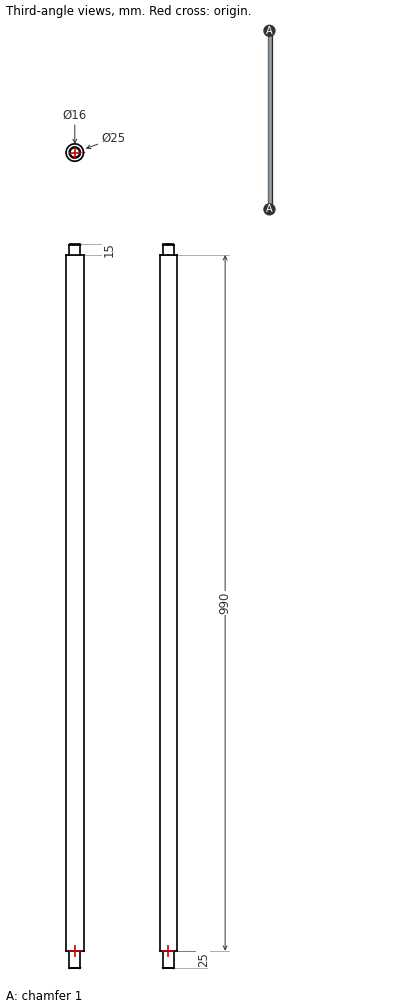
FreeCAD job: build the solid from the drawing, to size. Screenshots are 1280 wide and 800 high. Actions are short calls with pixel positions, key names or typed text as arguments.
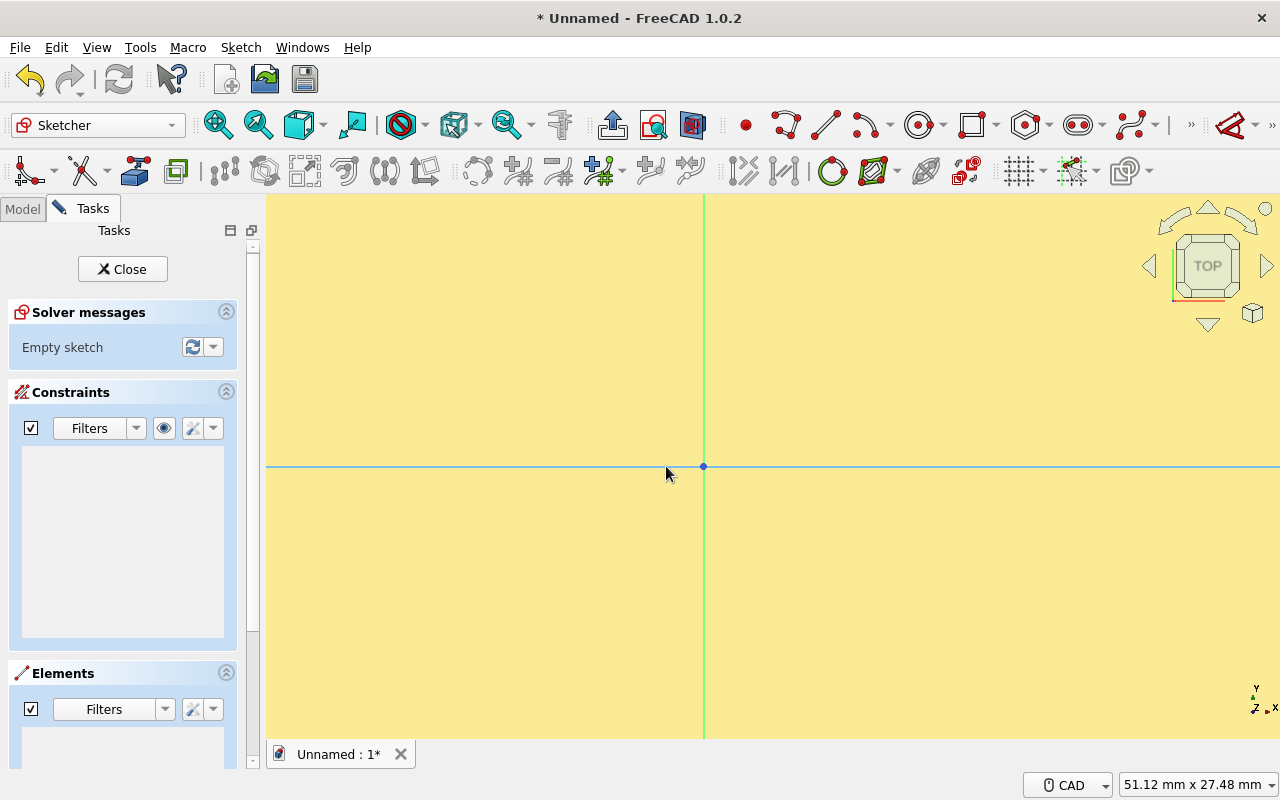
click(920, 126)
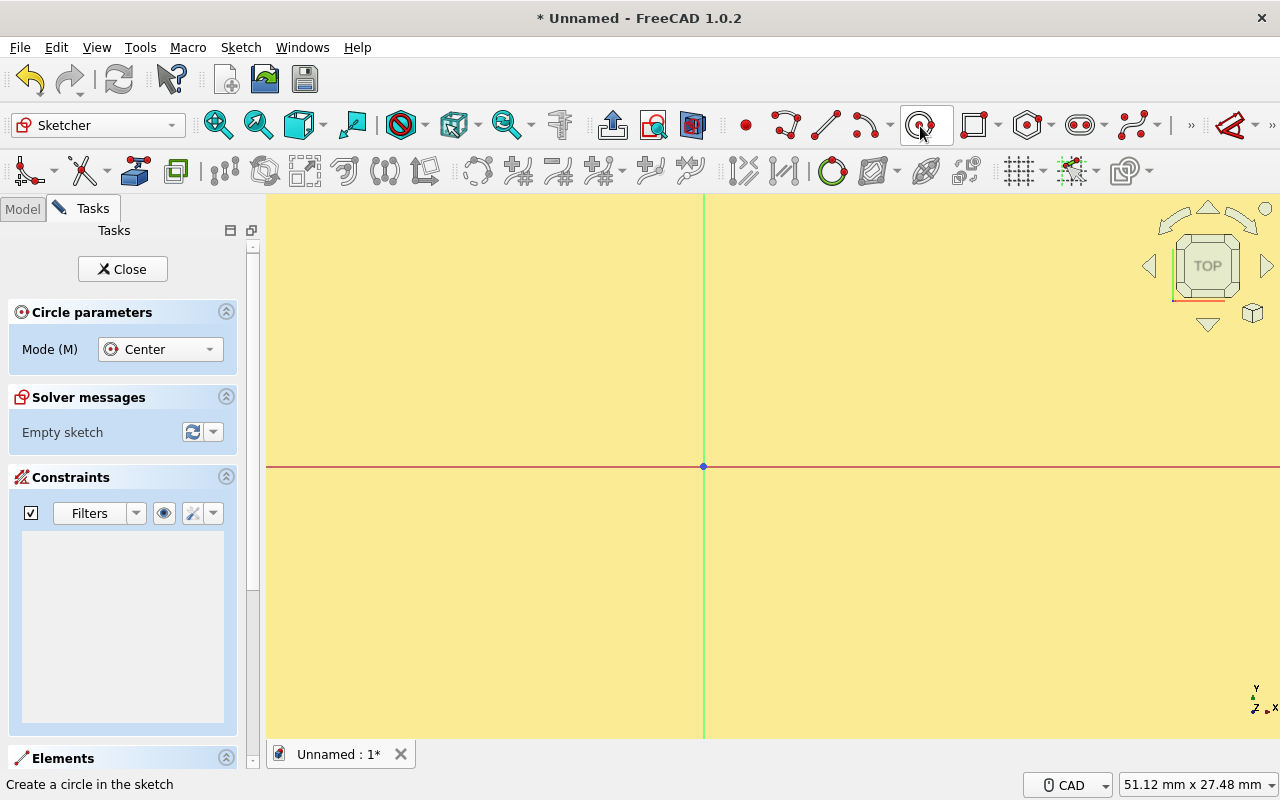
click(704, 466)
move(816, 354)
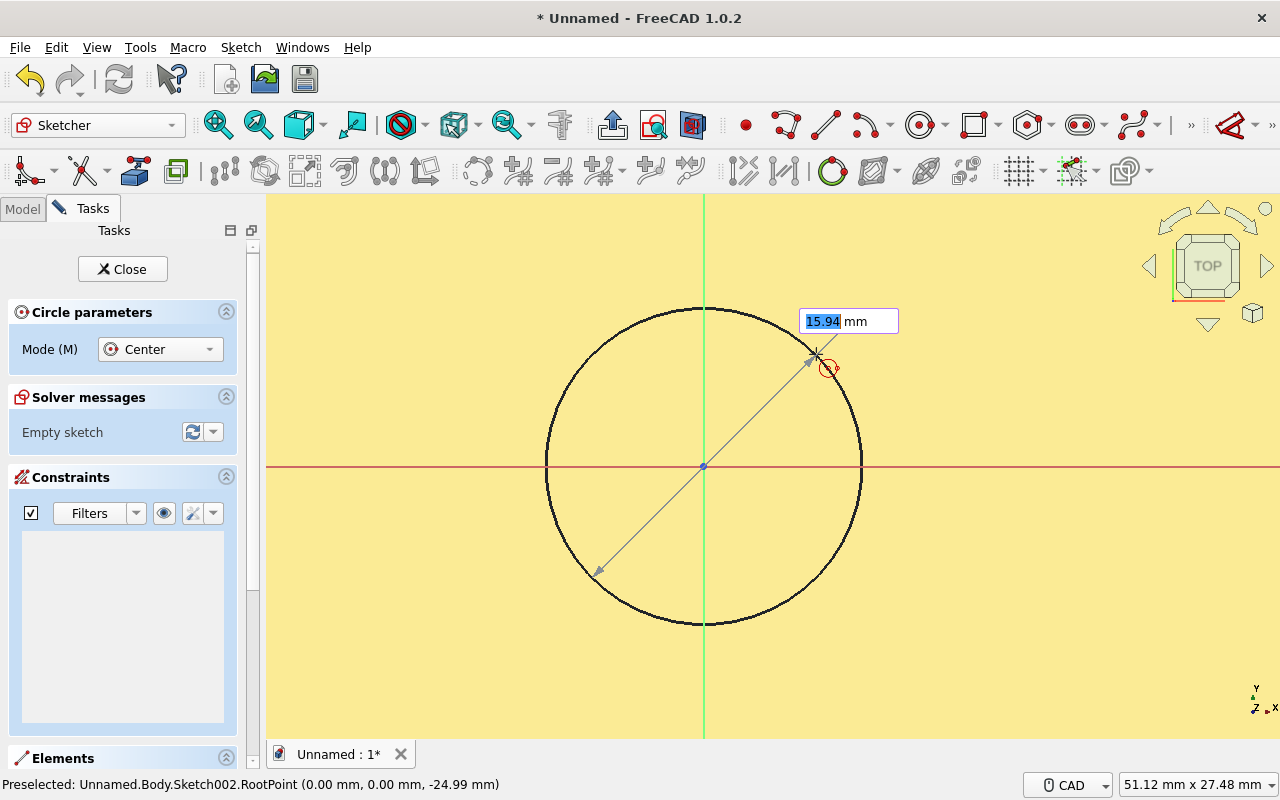
text(16)
key(Return)
key(Escape)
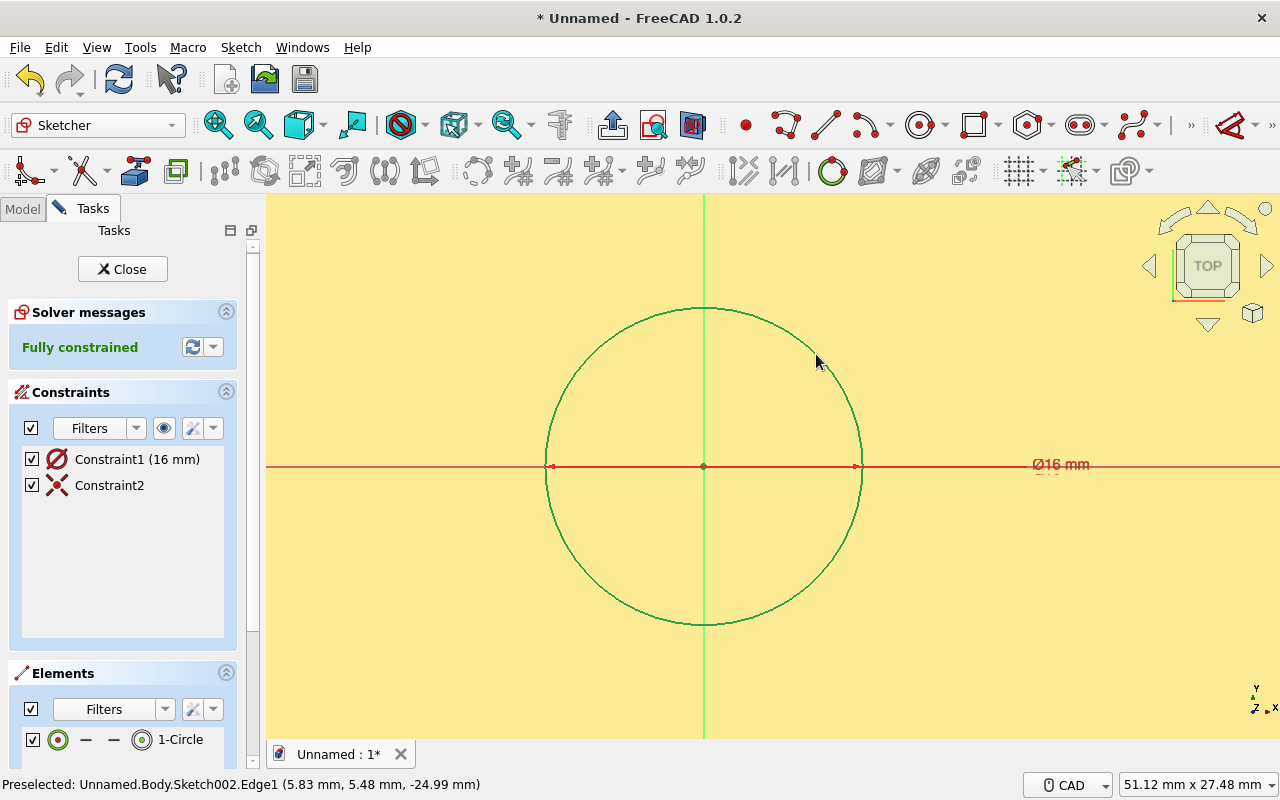
click(123, 269)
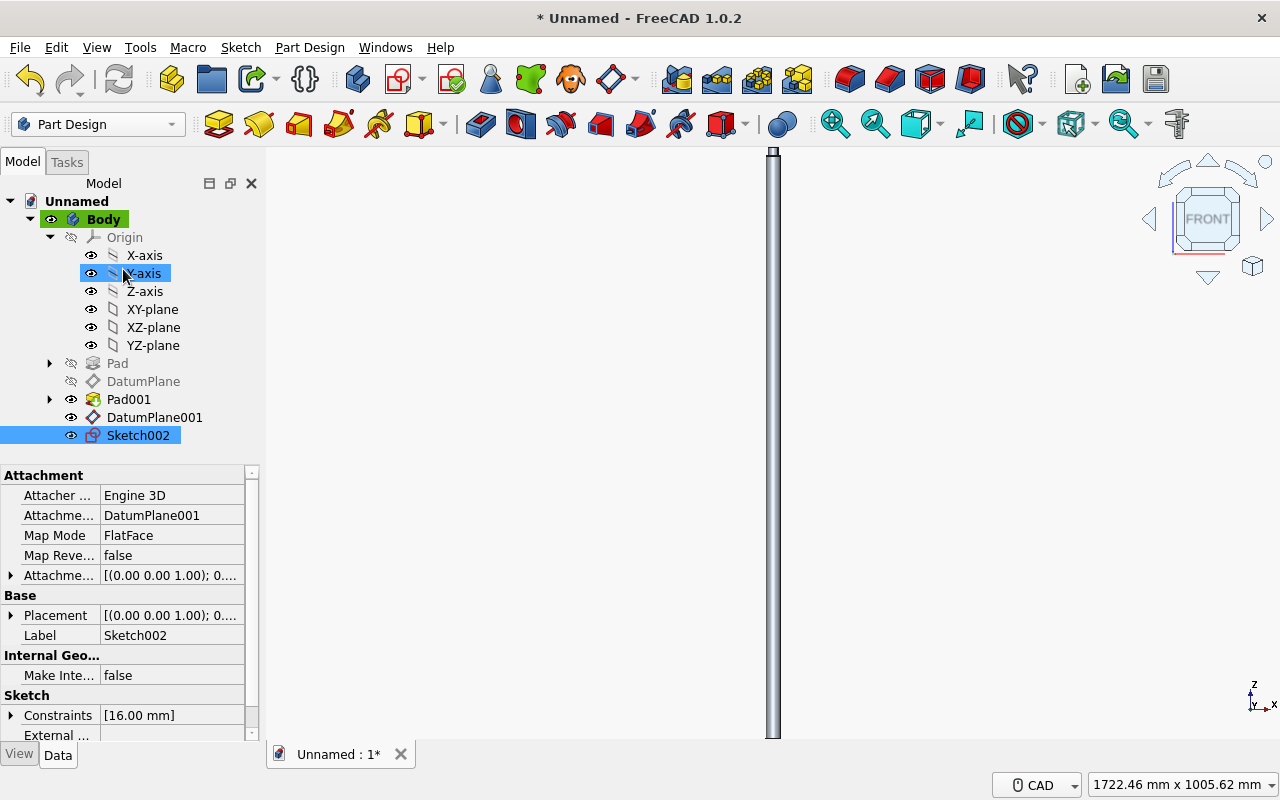
click(220, 124)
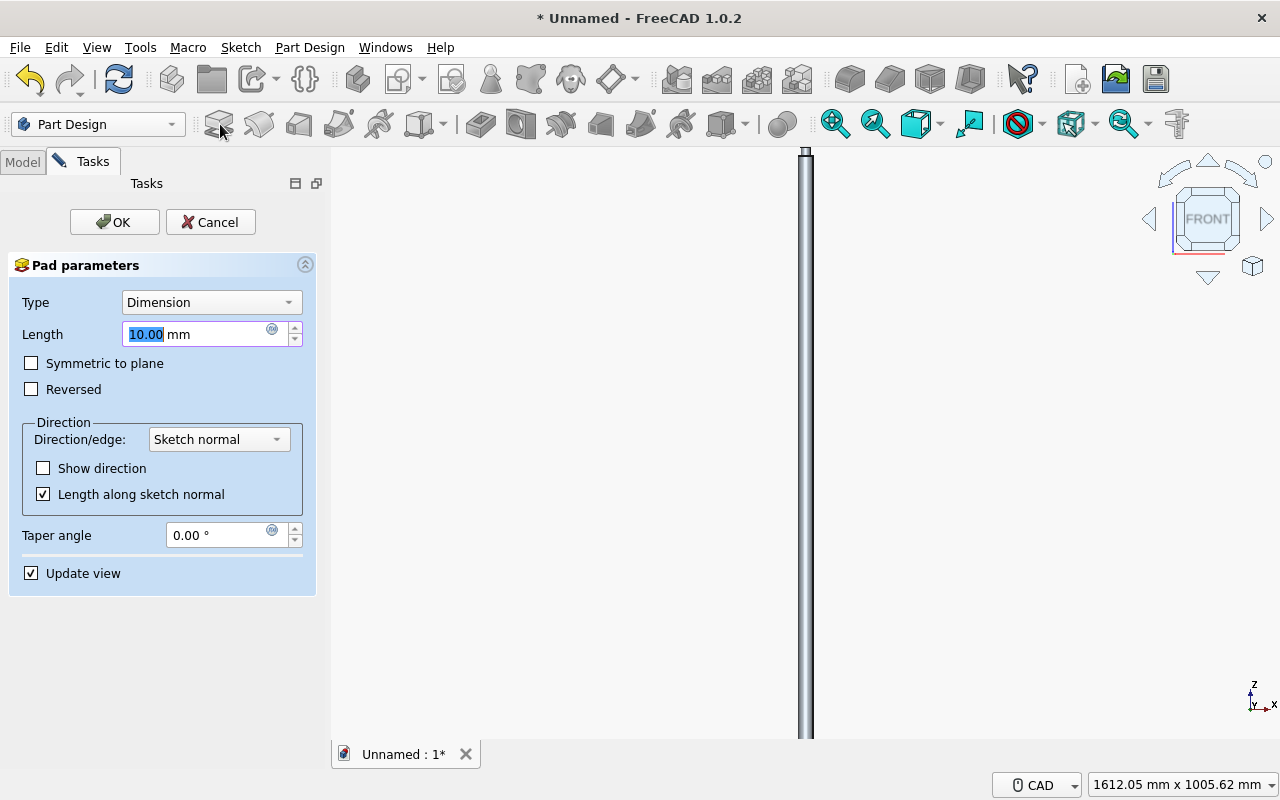
text(25)
key(Tab)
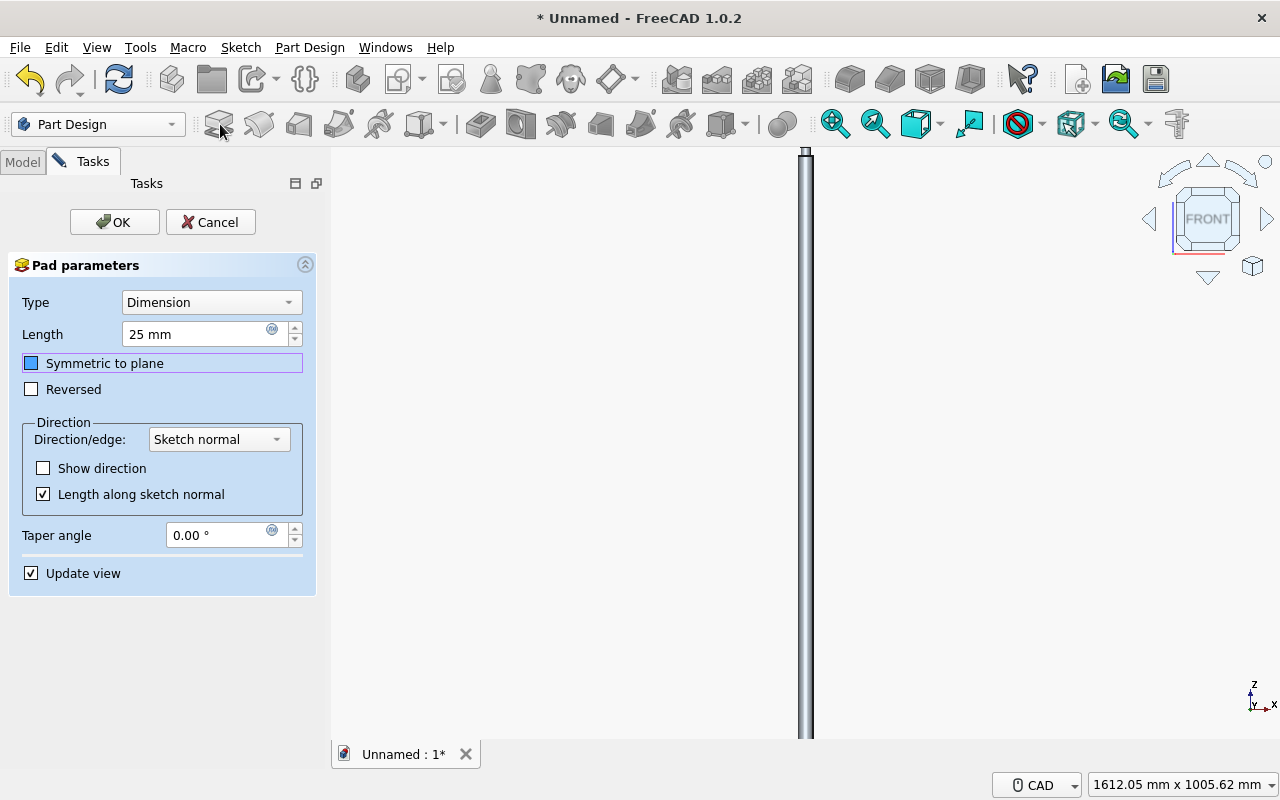
click(115, 222)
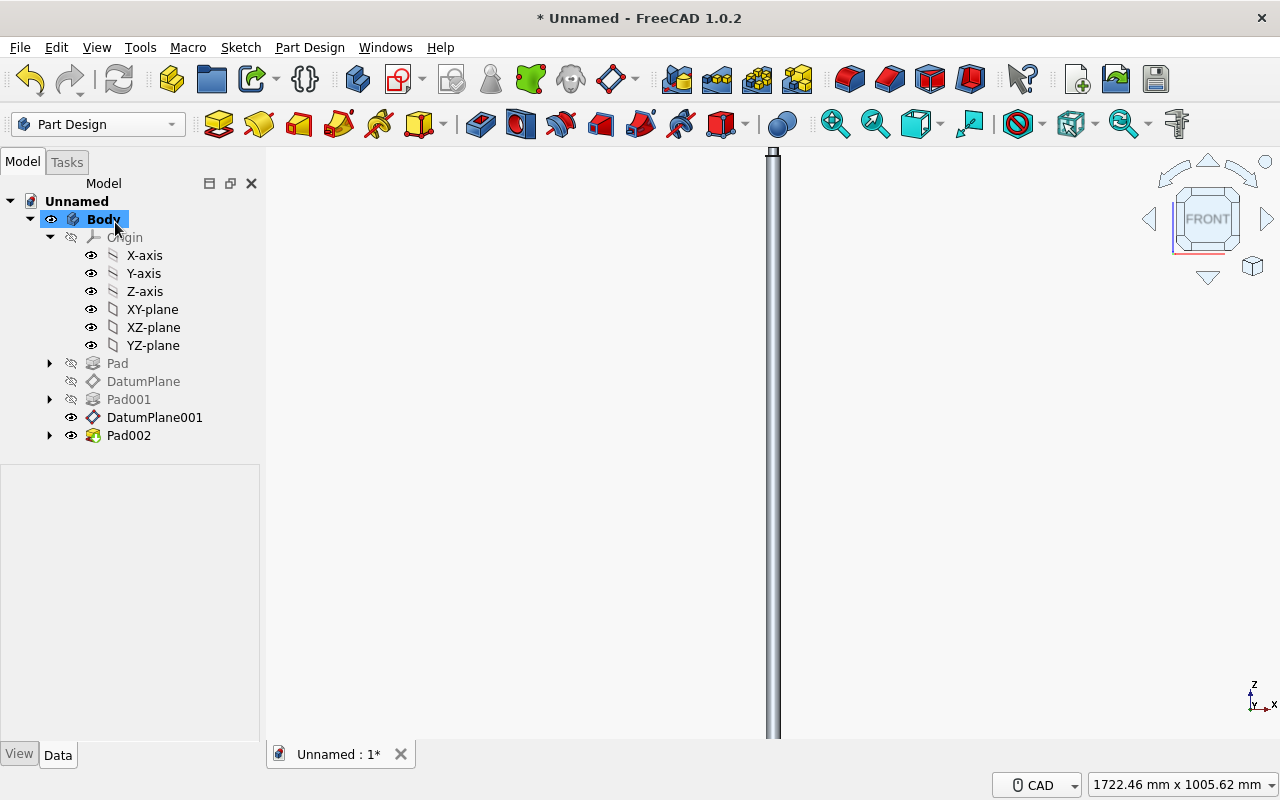
click(116, 417)
key(space)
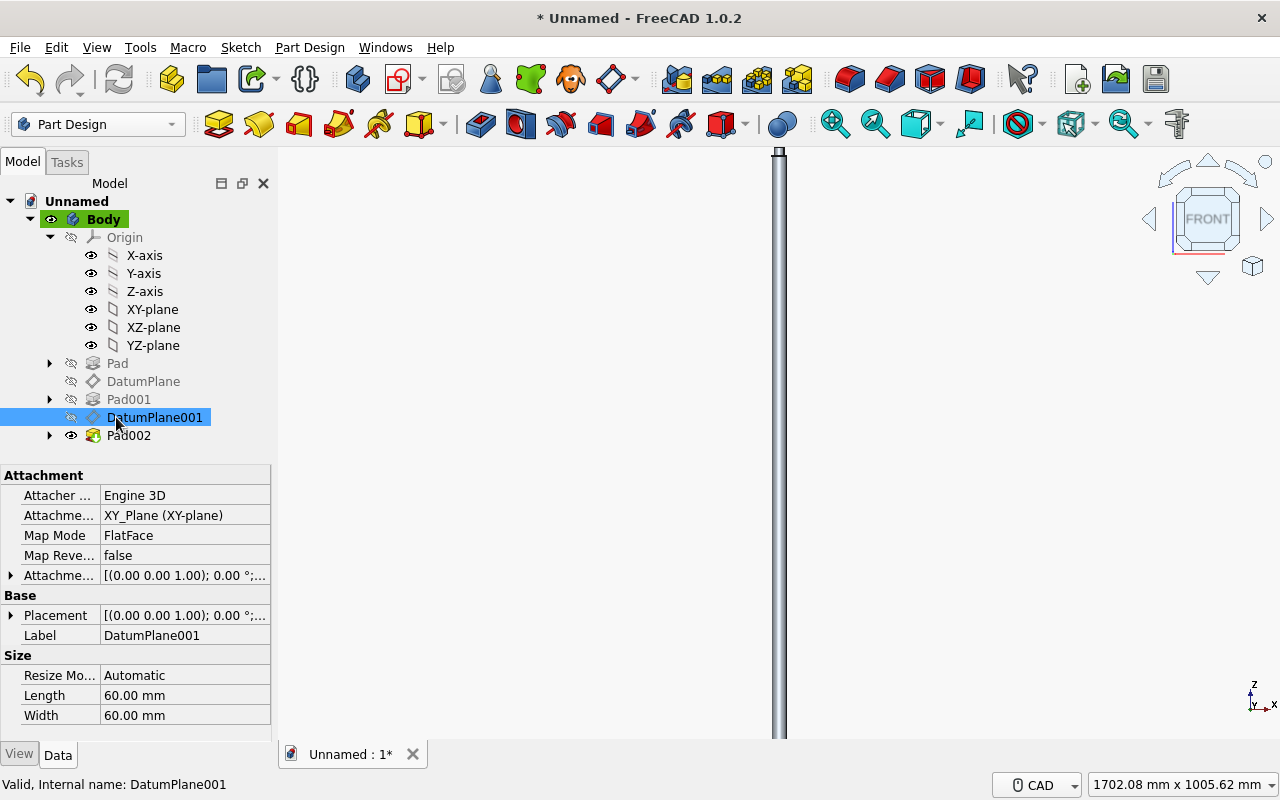
click(836, 124)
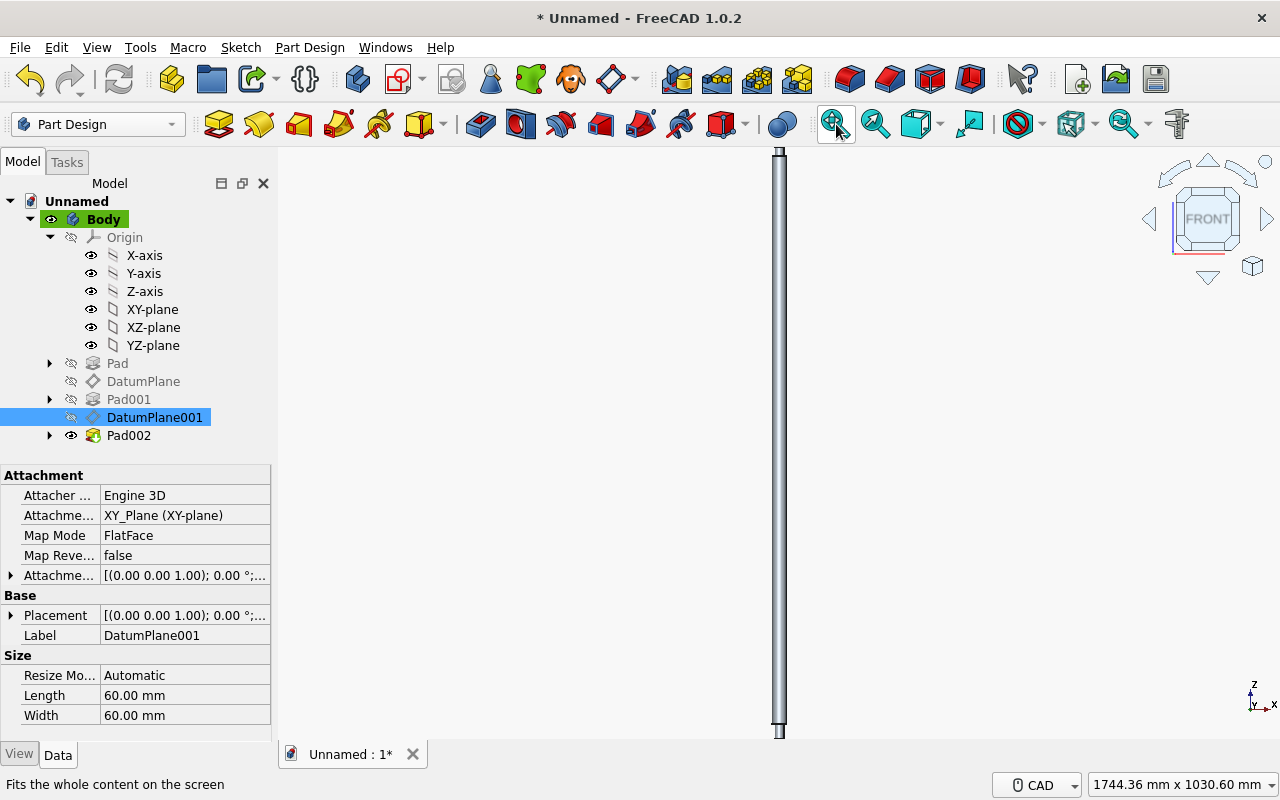
key(0)